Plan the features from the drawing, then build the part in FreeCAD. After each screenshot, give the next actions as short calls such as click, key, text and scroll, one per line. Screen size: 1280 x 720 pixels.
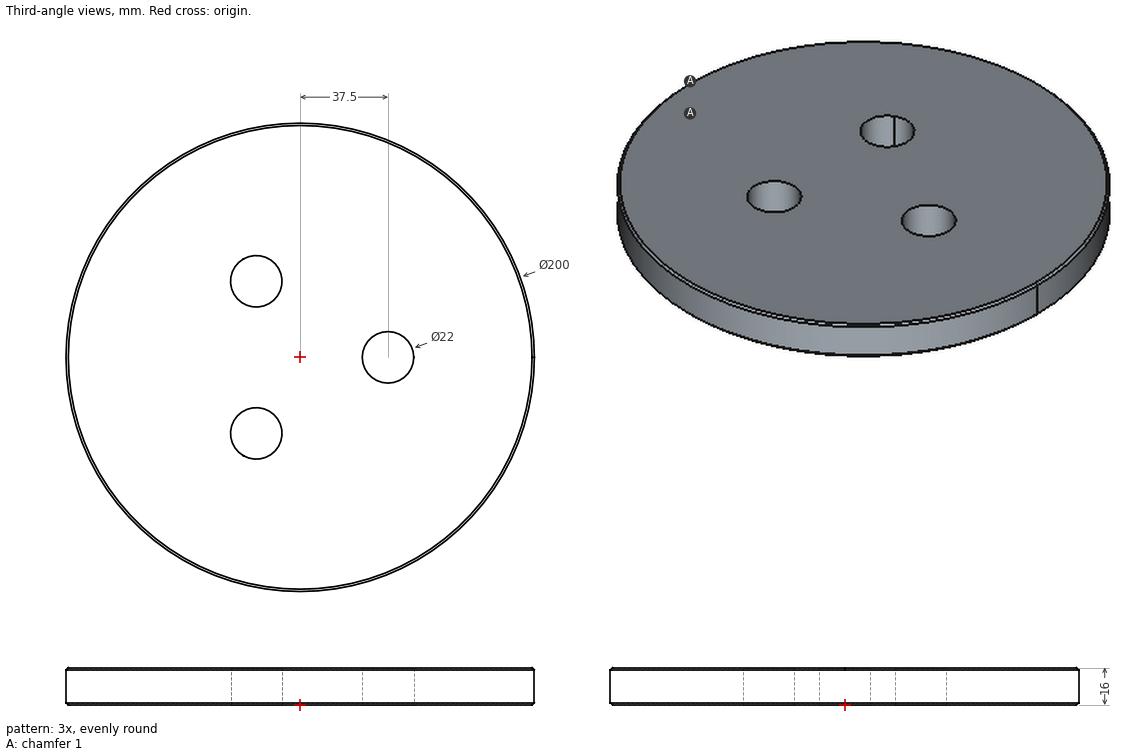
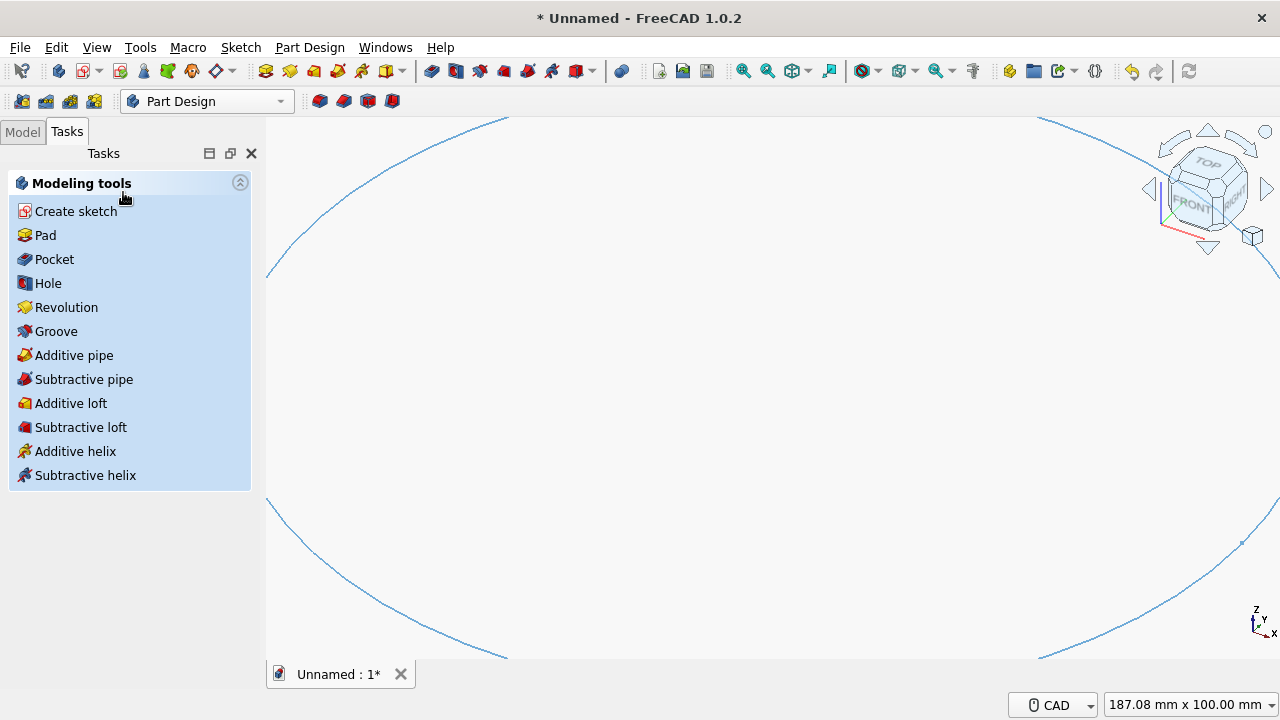
click(266, 72)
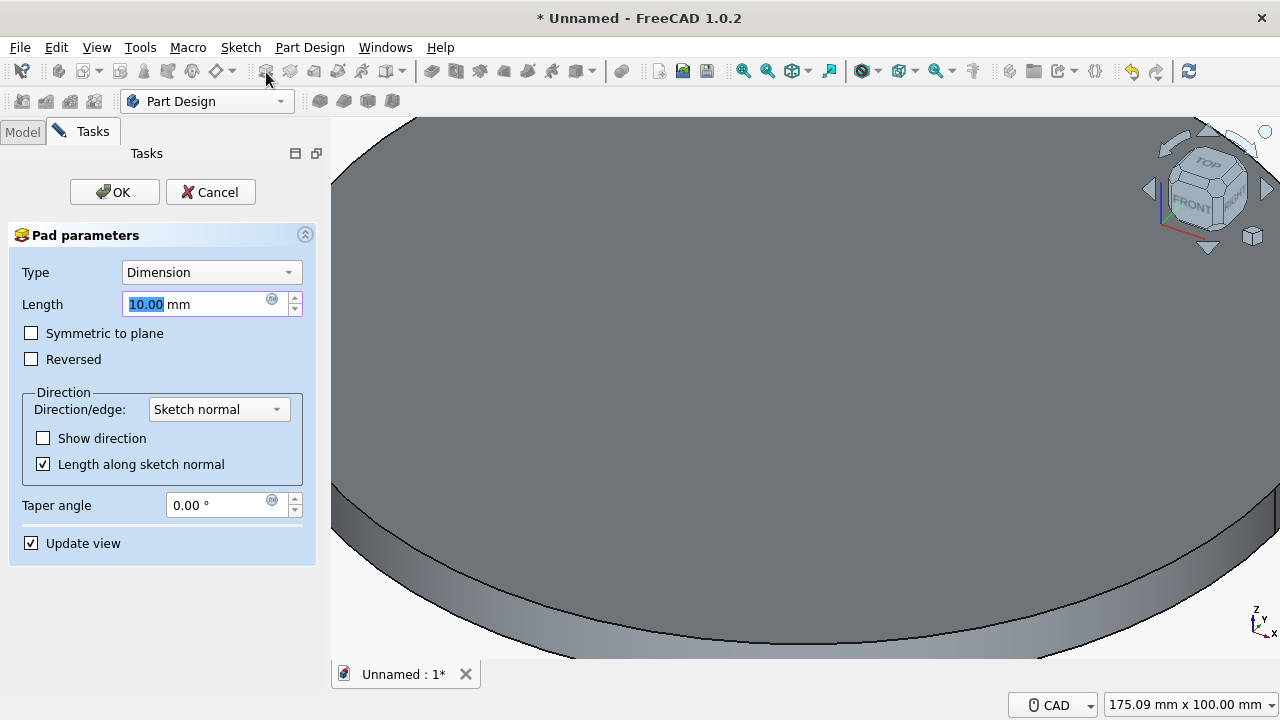
text(16)
key(Tab)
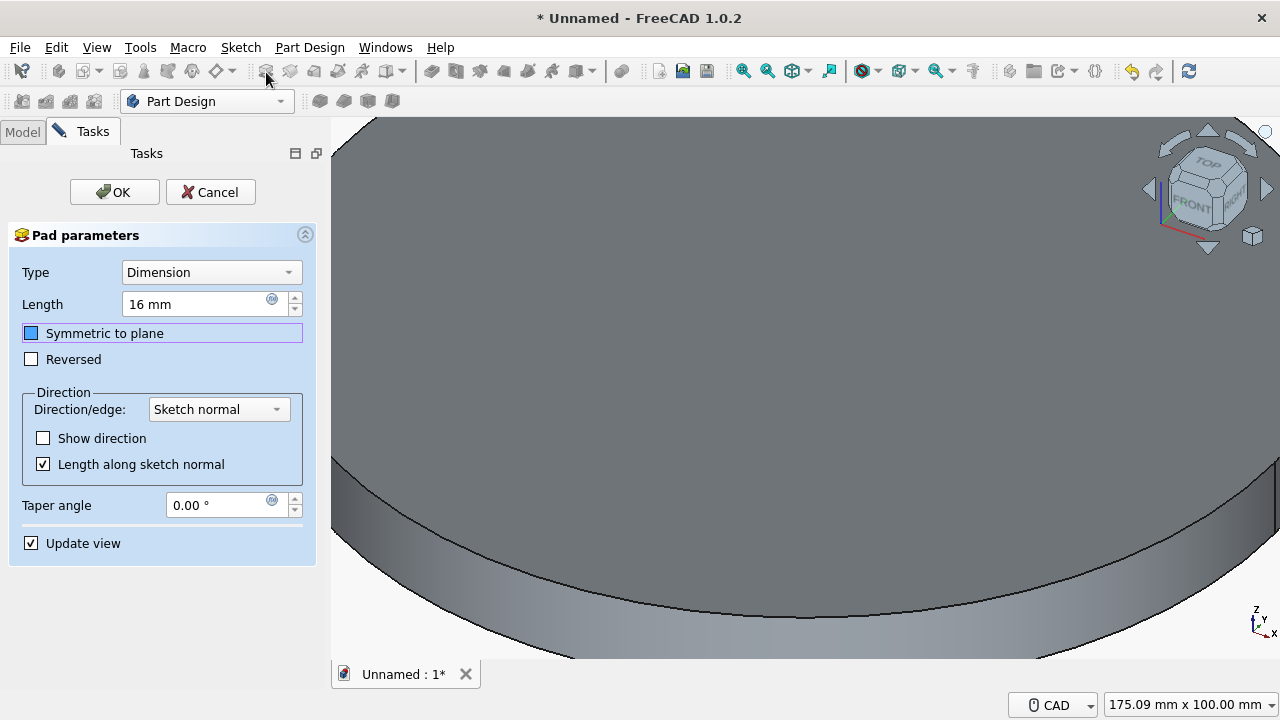
click(115, 192)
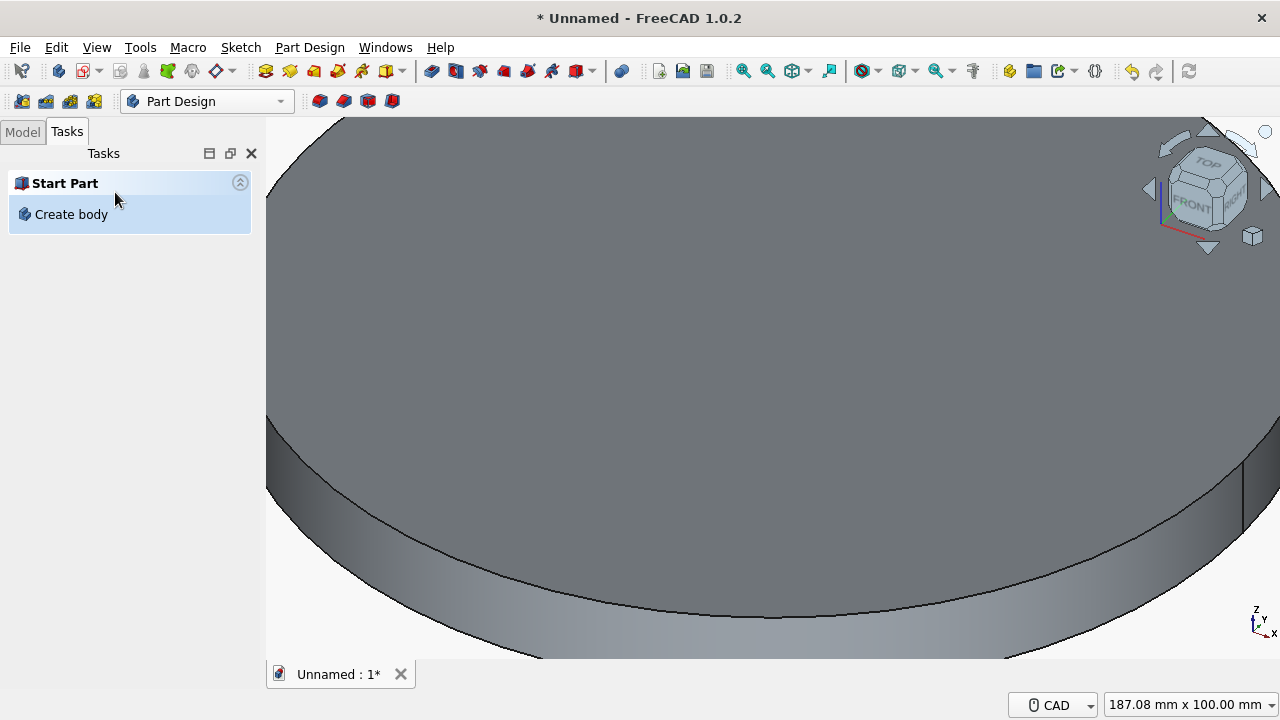
click(744, 72)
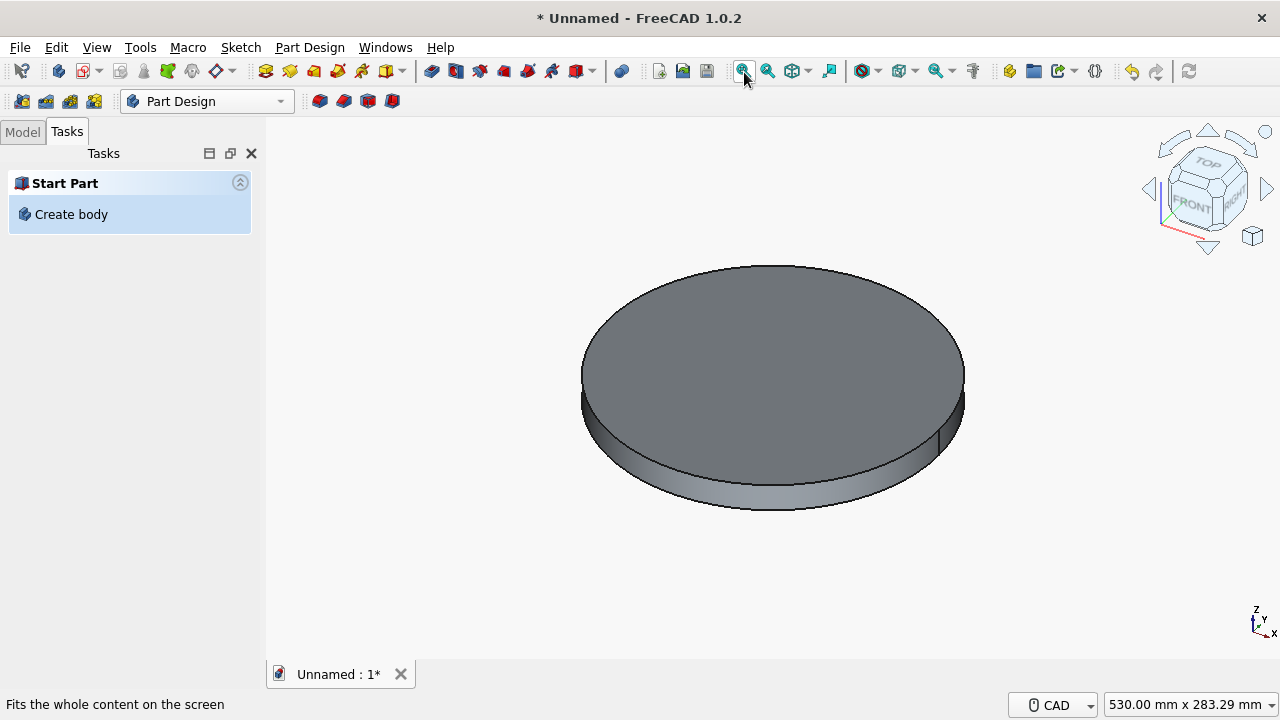
click(773, 374)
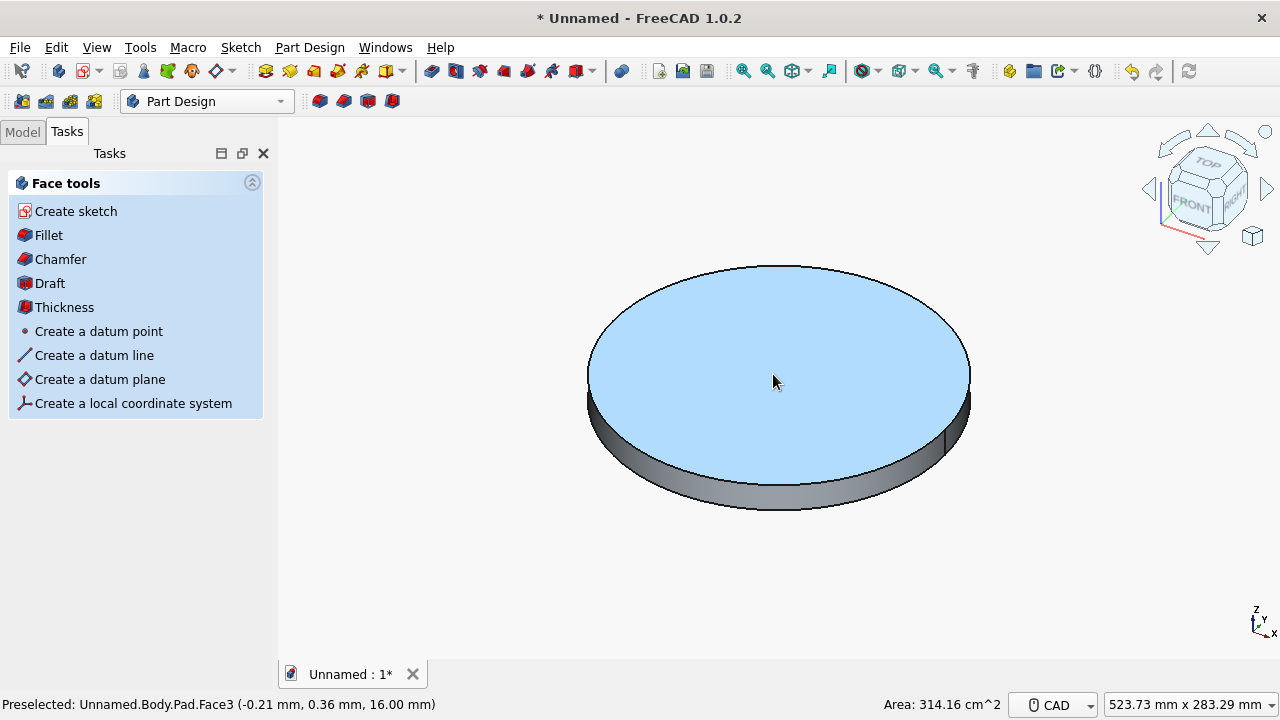
click(84, 72)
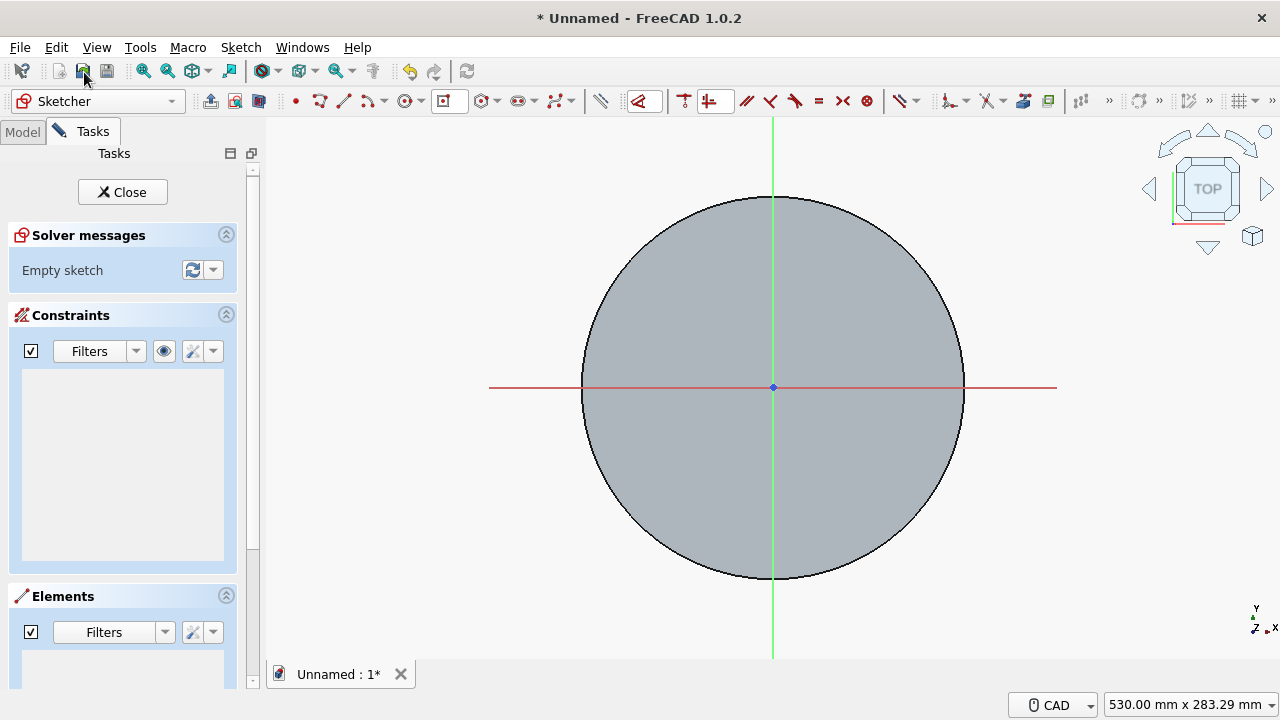
scroll(842, 388, up, 9)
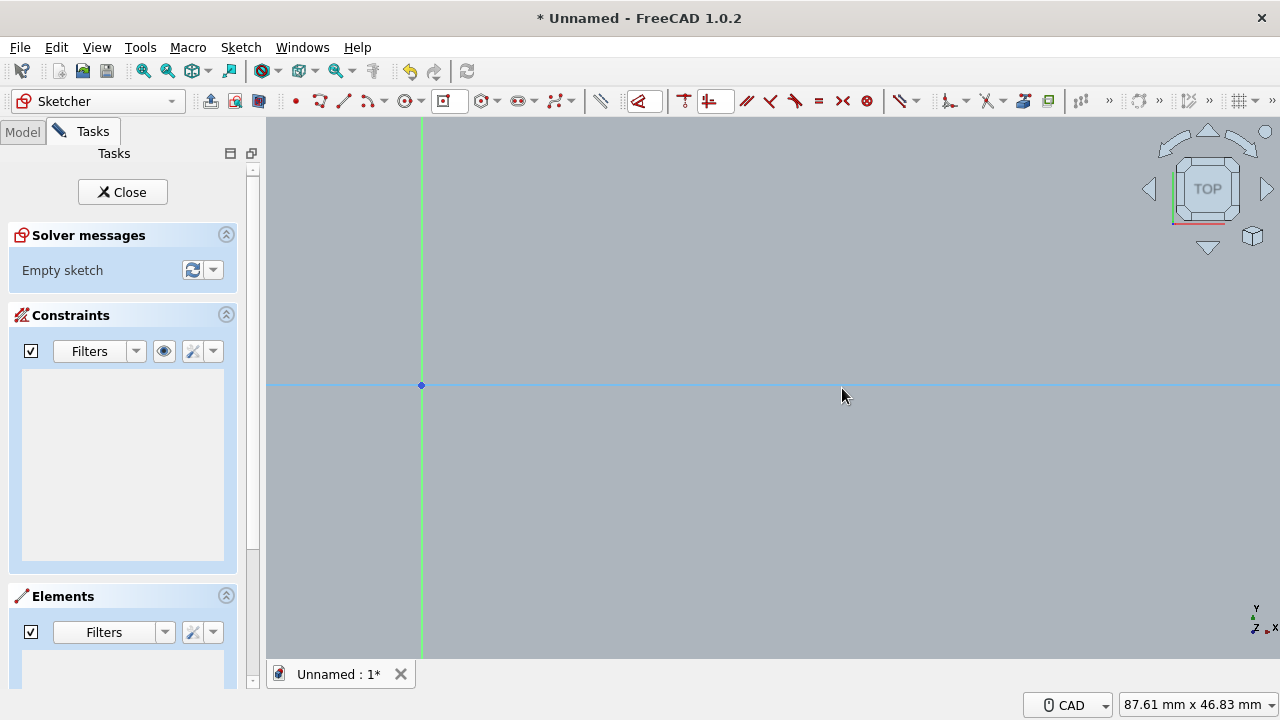
click(406, 102)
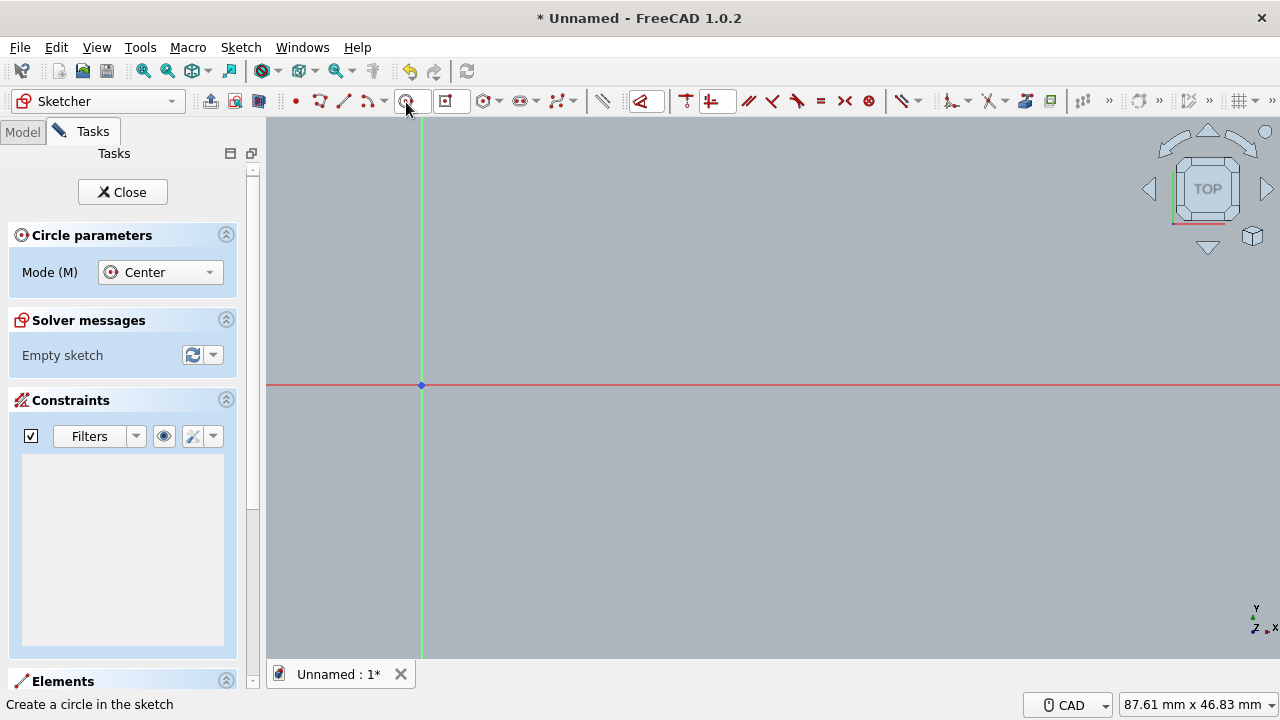
click(856, 385)
click(946, 295)
key(Escape)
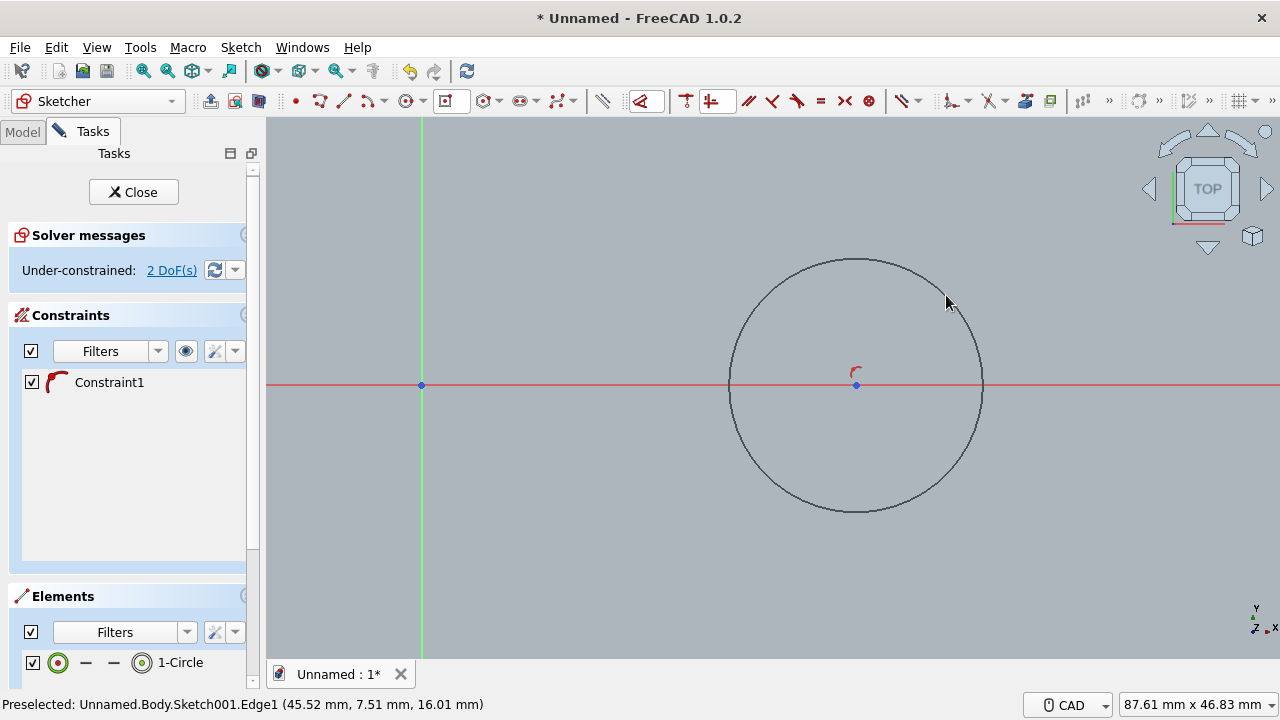
click(640, 102)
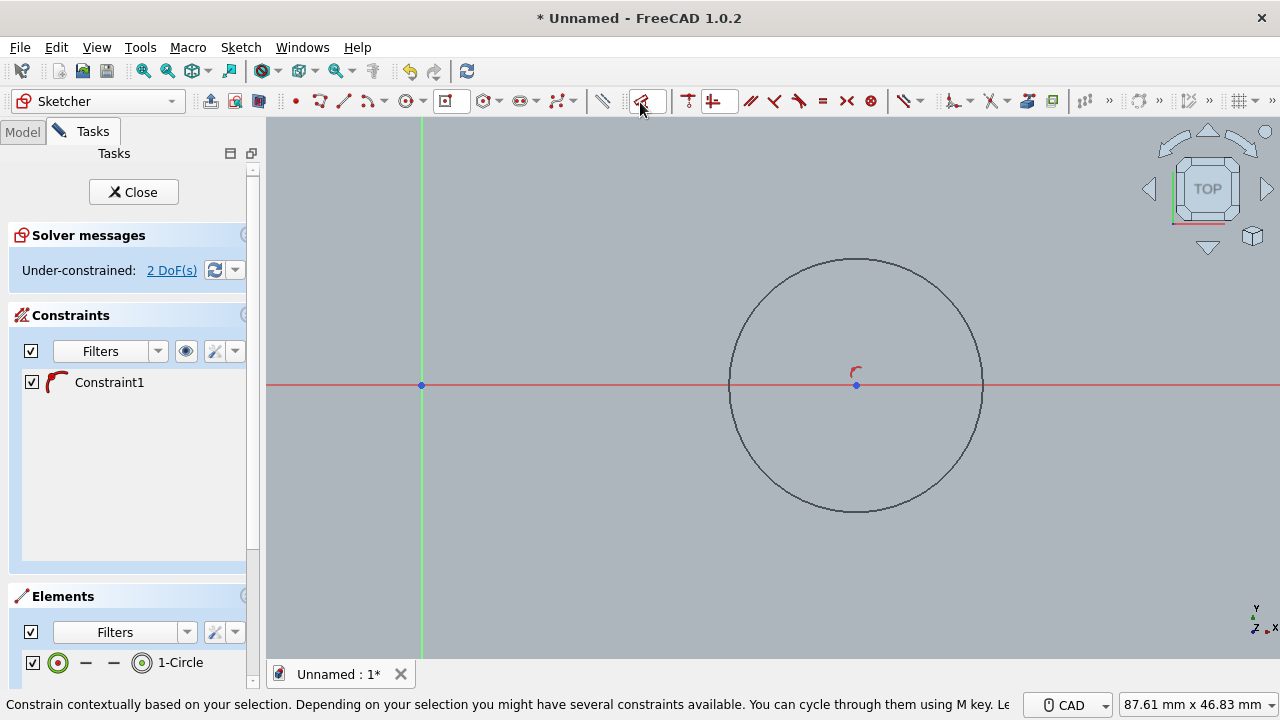
click(945, 295)
click(967, 272)